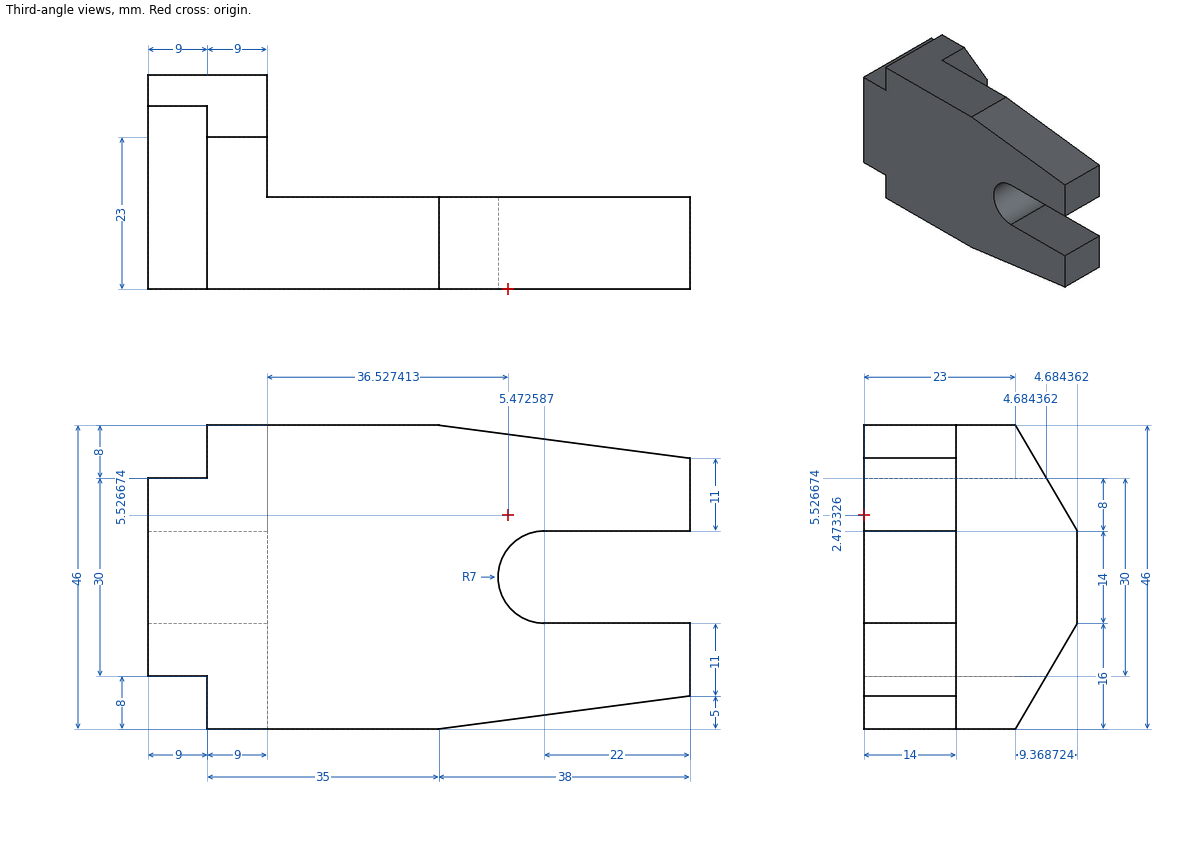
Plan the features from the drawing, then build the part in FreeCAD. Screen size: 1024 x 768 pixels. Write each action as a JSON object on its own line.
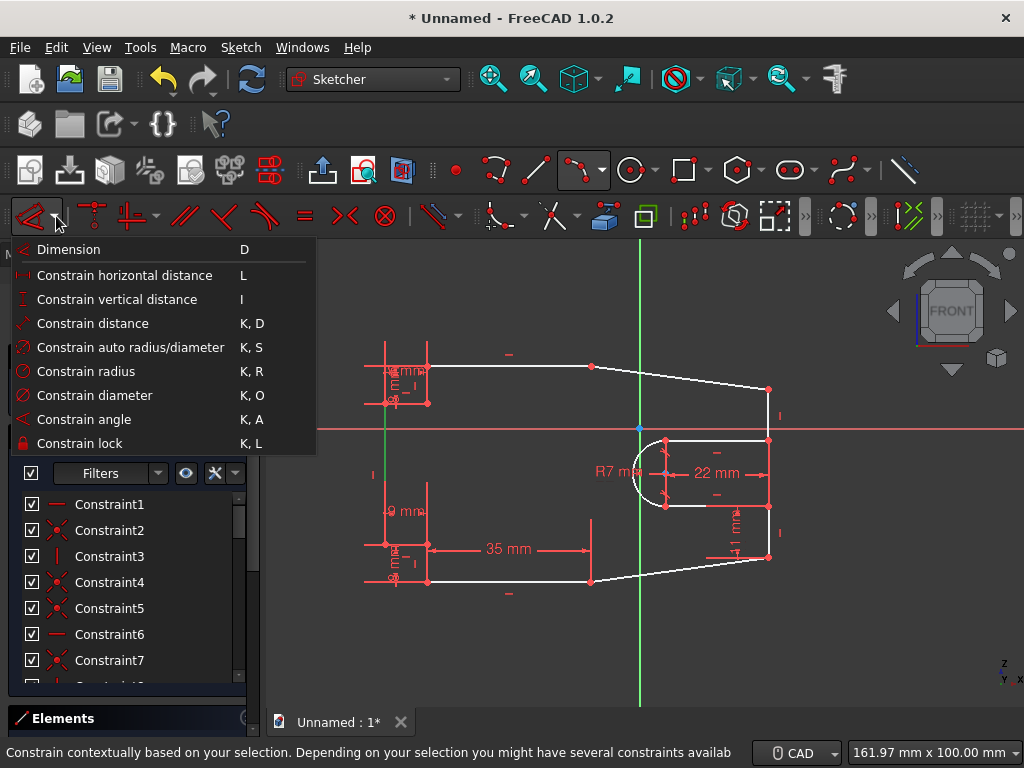
{"action": "left_click", "coordinate": [164, 299]}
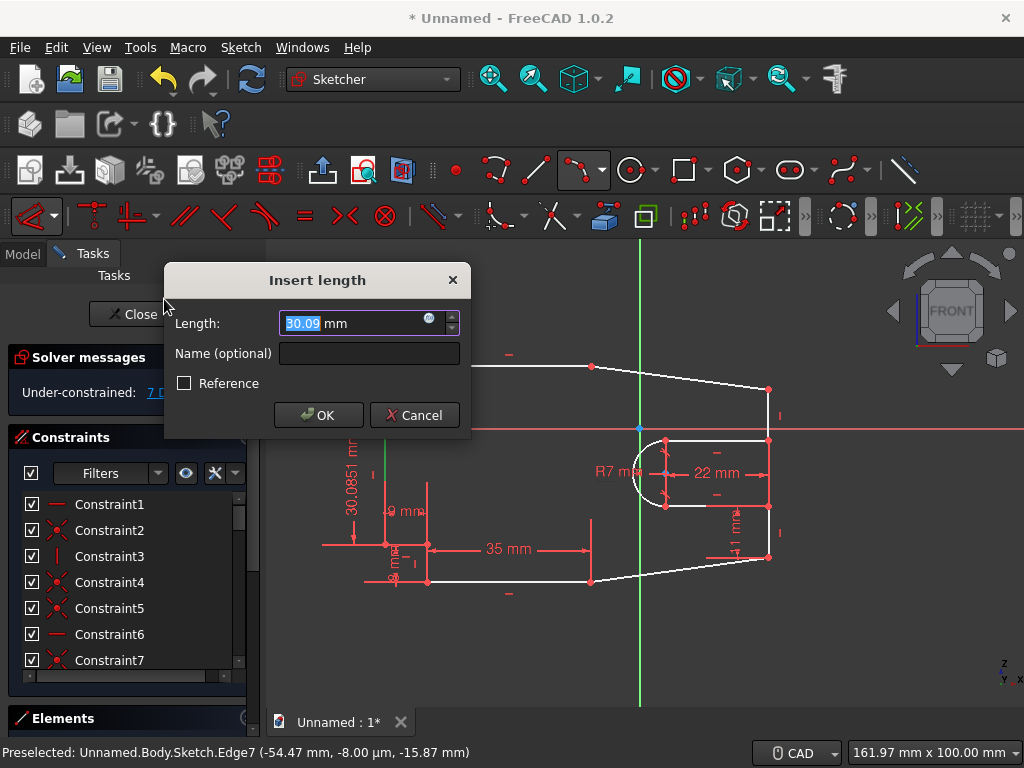
{"action": "type", "text": "30"}
{"action": "key", "text": "Return"}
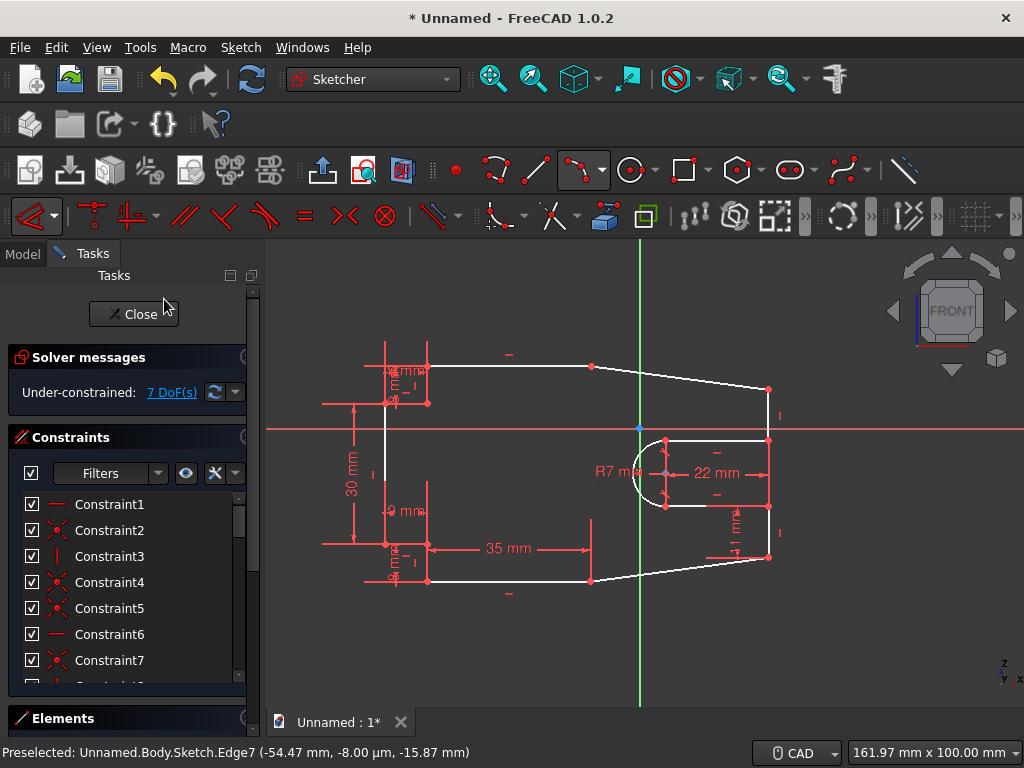
{"action": "left_click", "coordinate": [476, 366]}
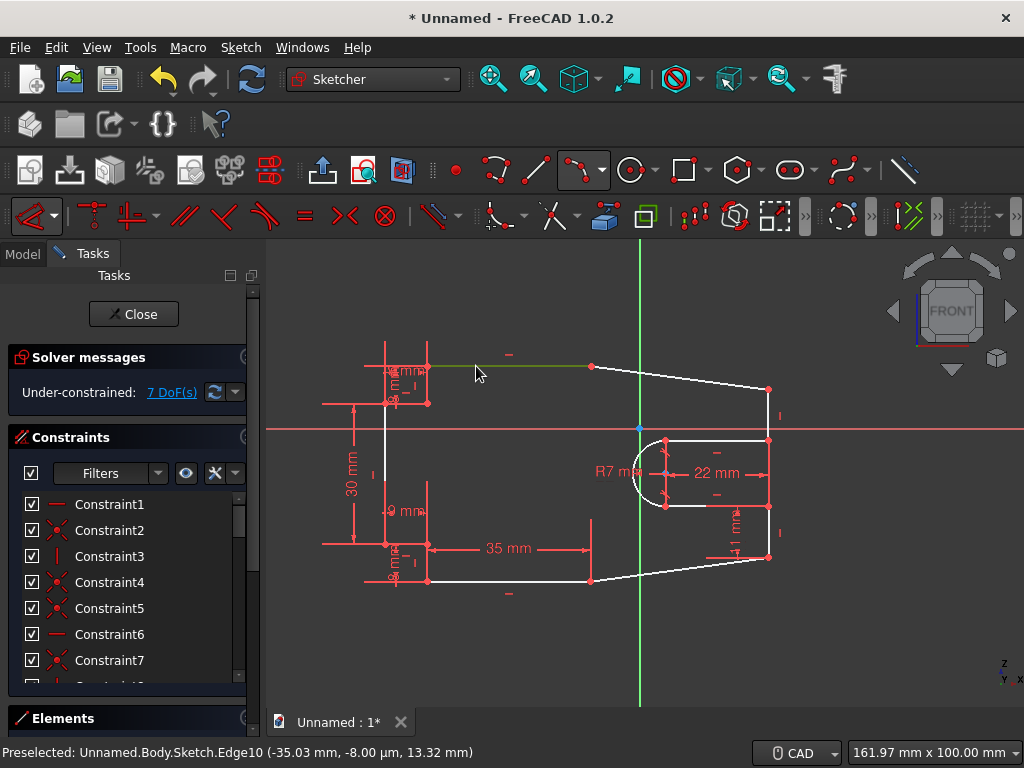
{"action": "key", "text": "l"}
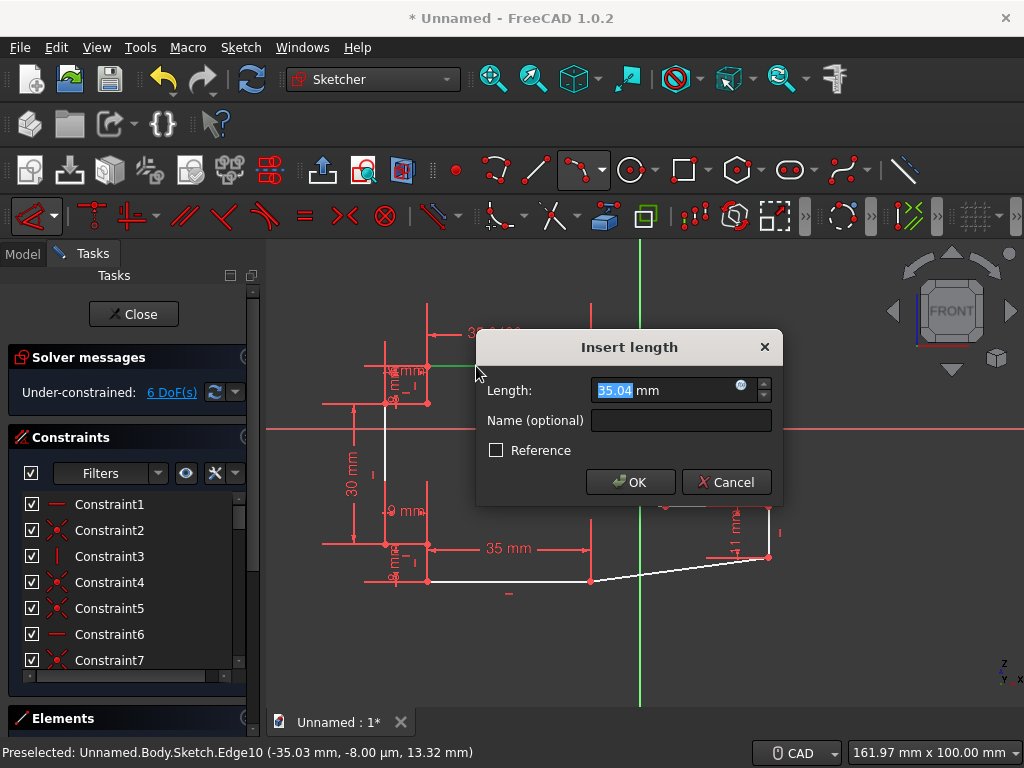
{"action": "type", "text": "35"}
{"action": "key", "text": "Return"}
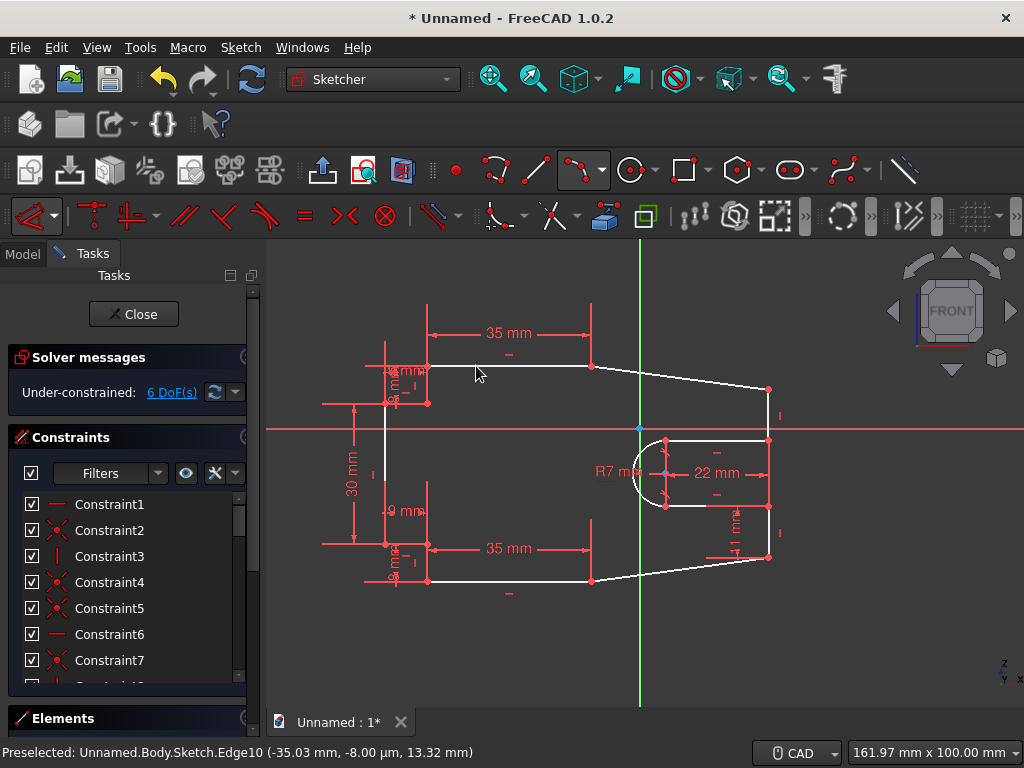
{"action": "left_click", "coordinate": [768, 405]}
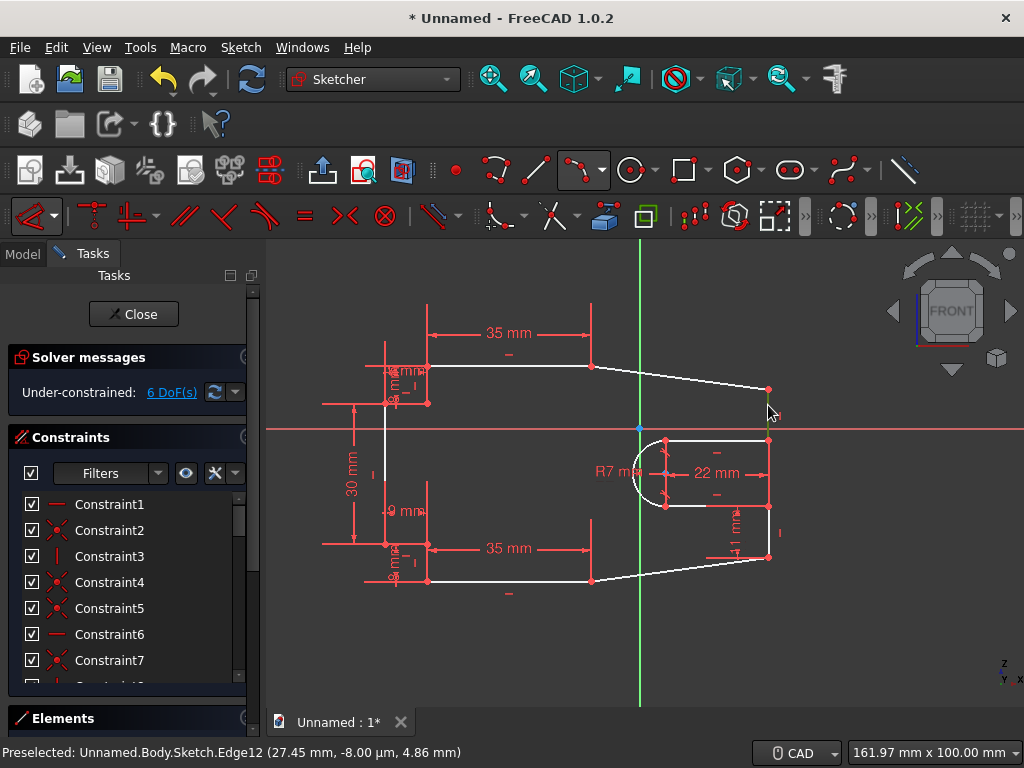
{"action": "left_click", "coordinate": [56, 216]}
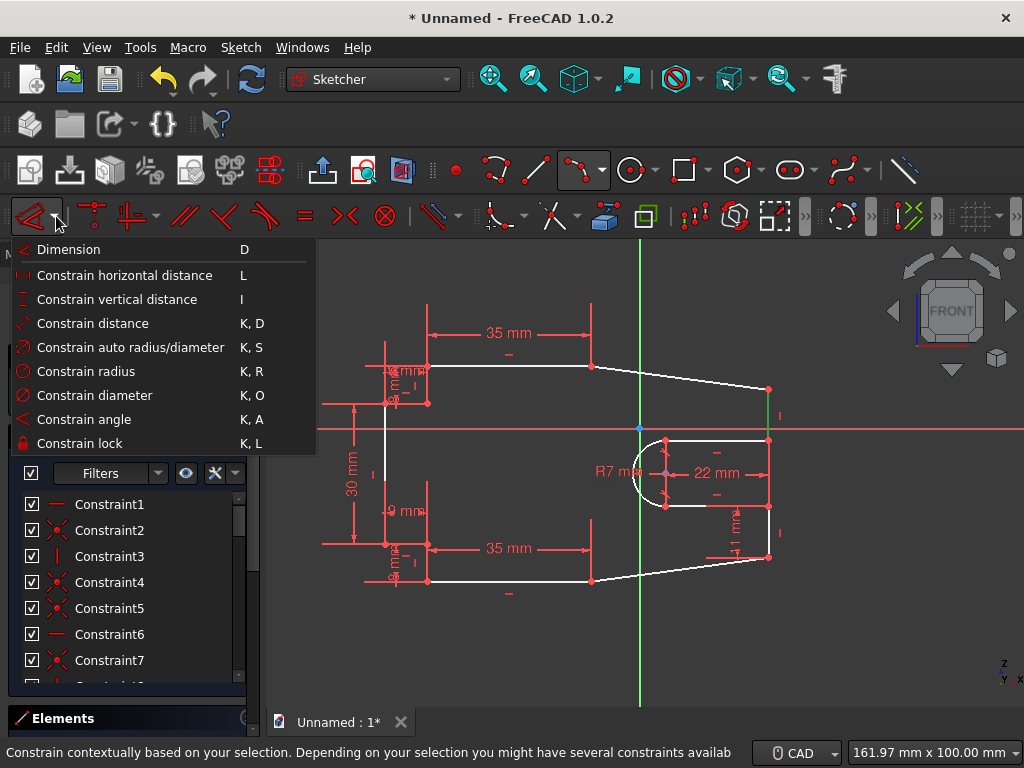
{"action": "left_click", "coordinate": [164, 299]}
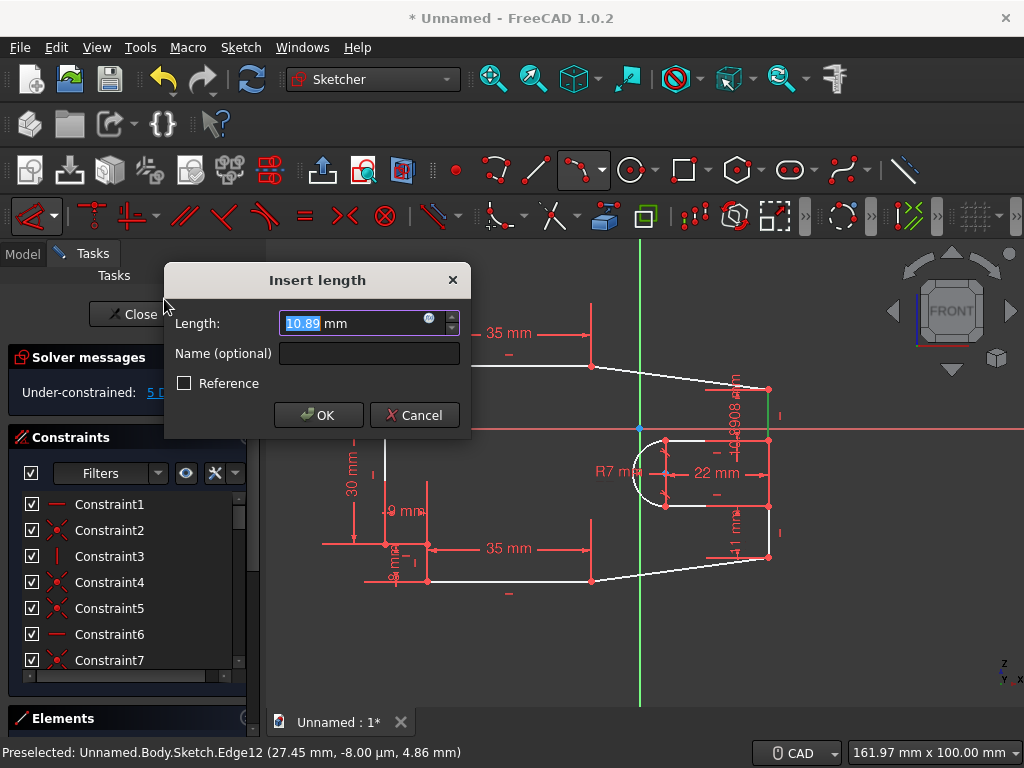
{"action": "type", "text": "11"}
{"action": "key", "text": "Return"}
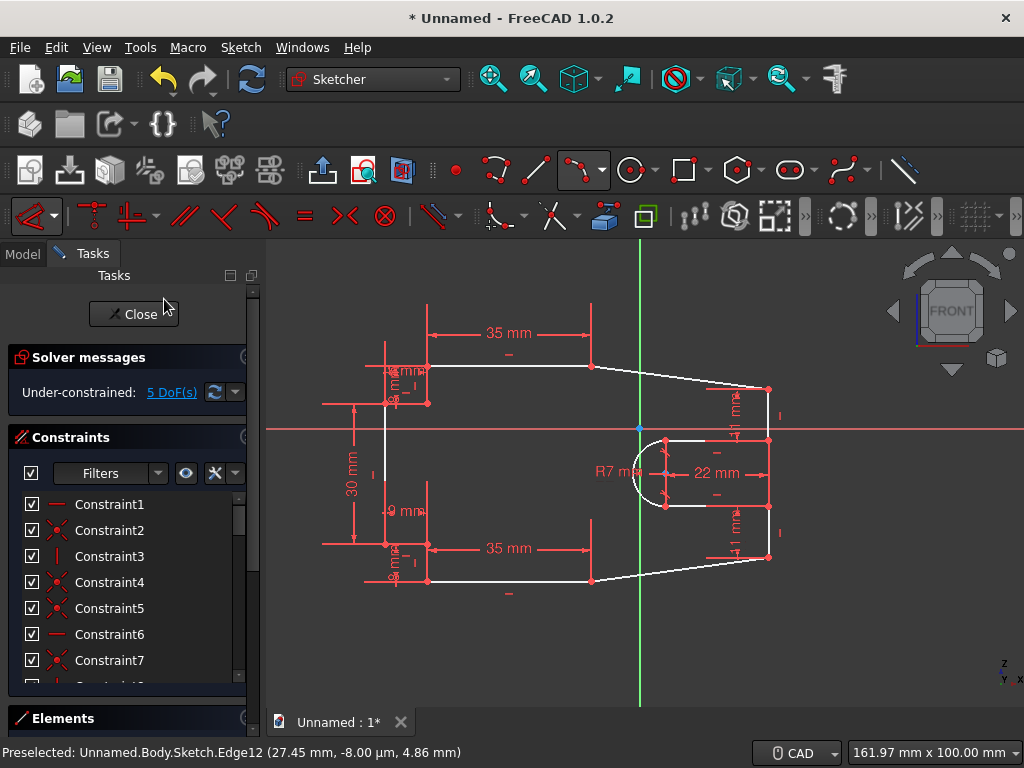
{"action": "left_click", "coordinate": [738, 441]}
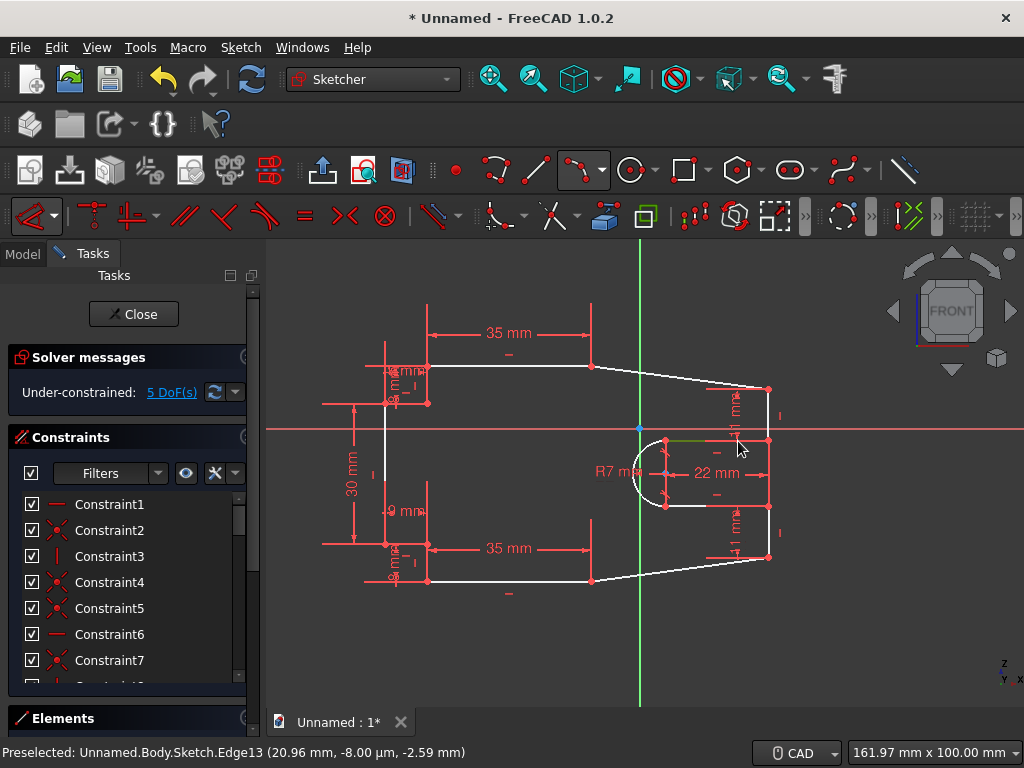
{"action": "key", "text": "l"}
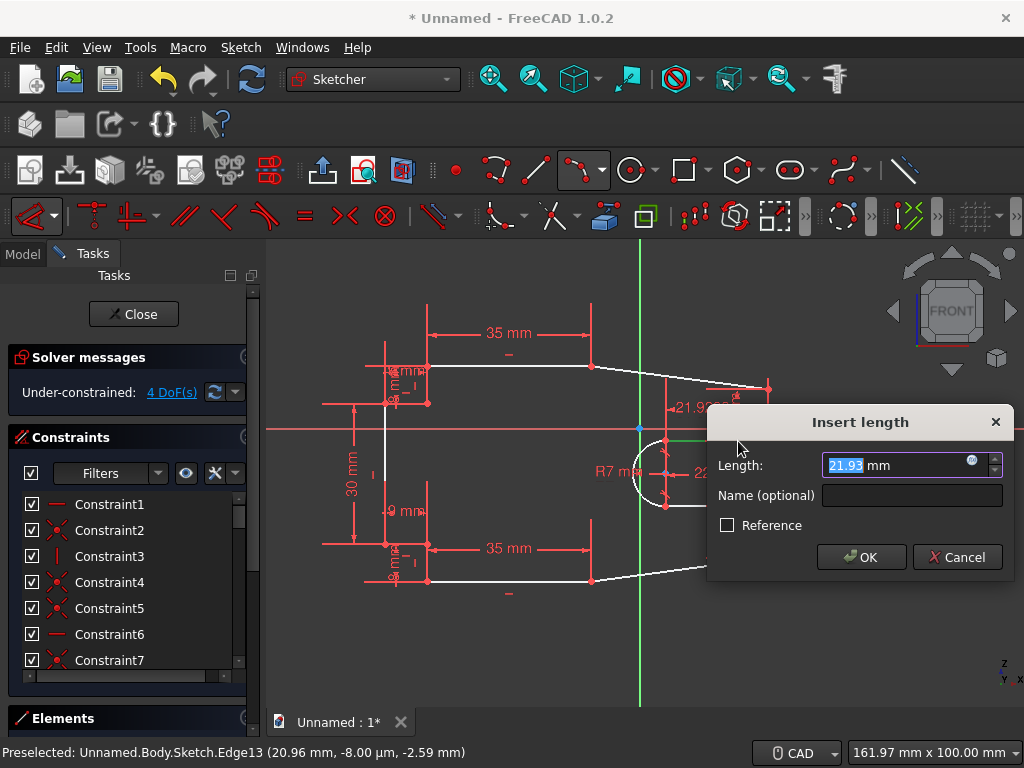
{"action": "type", "text": "22"}
{"action": "key", "text": "Return"}